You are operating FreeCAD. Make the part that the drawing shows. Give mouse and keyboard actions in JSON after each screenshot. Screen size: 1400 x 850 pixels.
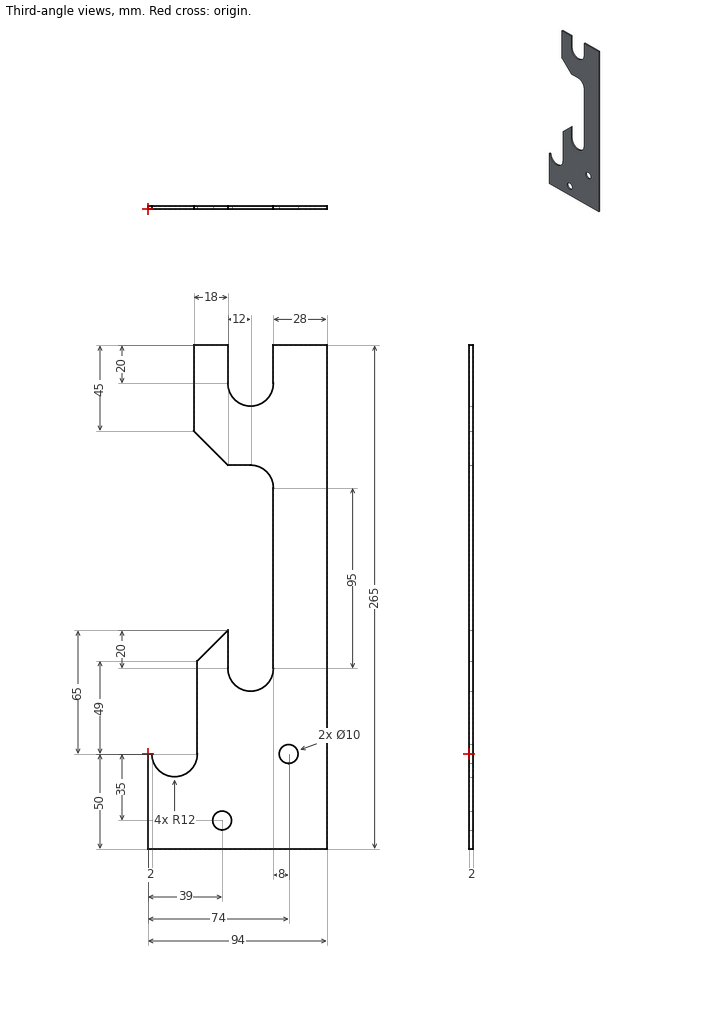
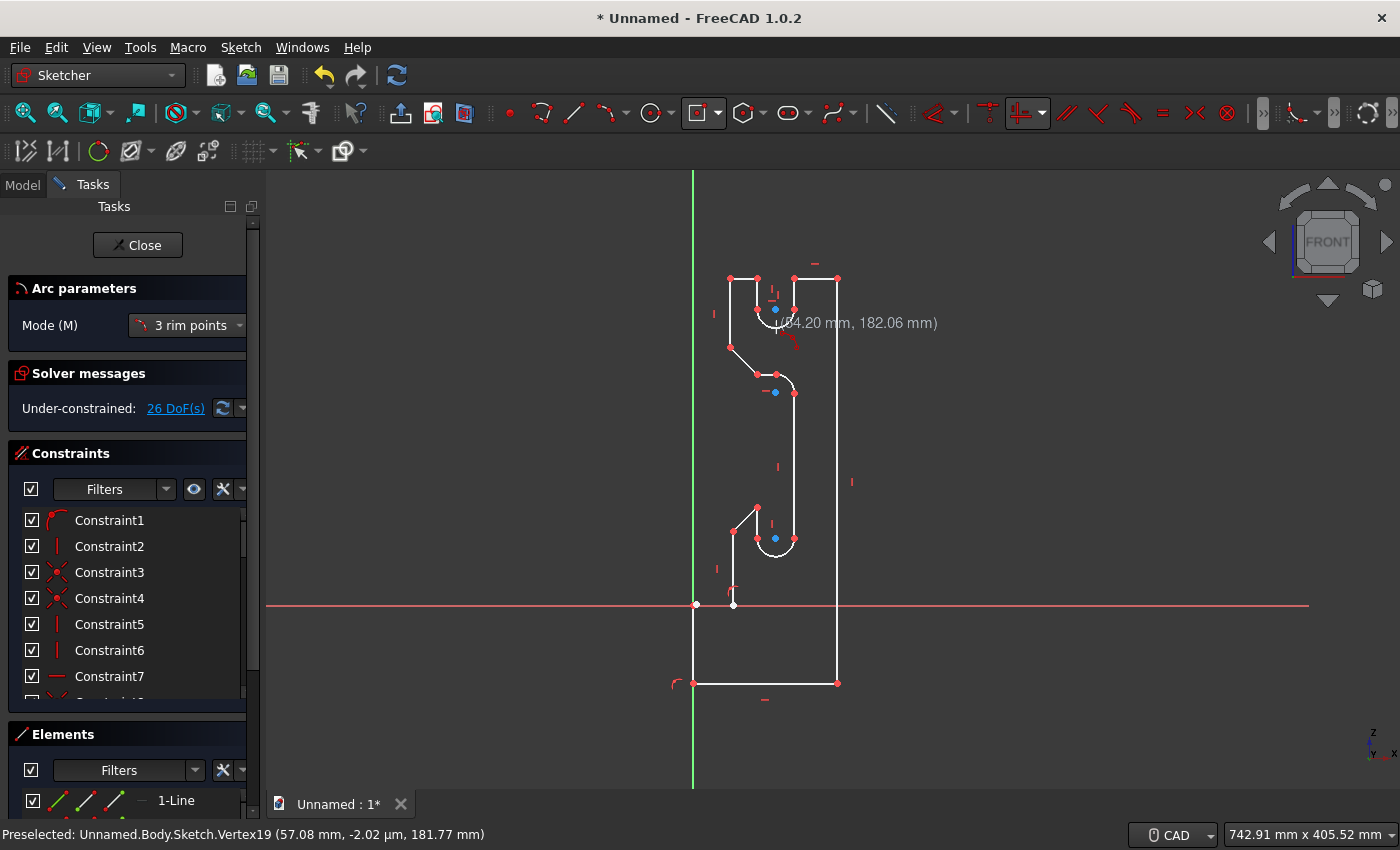
{"action": "scroll", "coordinate": [696, 606], "scroll_direction": "up", "scroll_amount": 12}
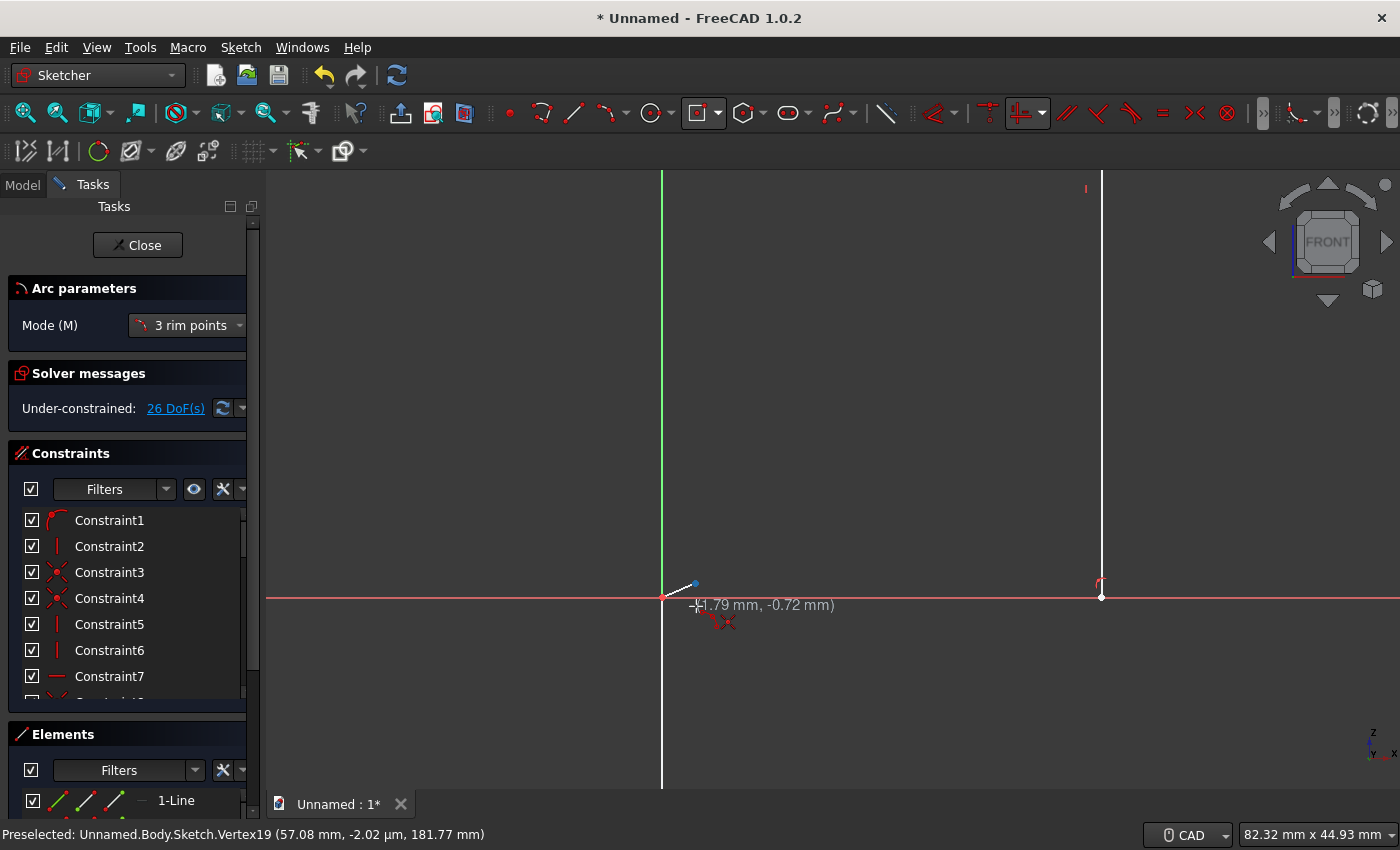
{"action": "left_click", "coordinate": [695, 583]}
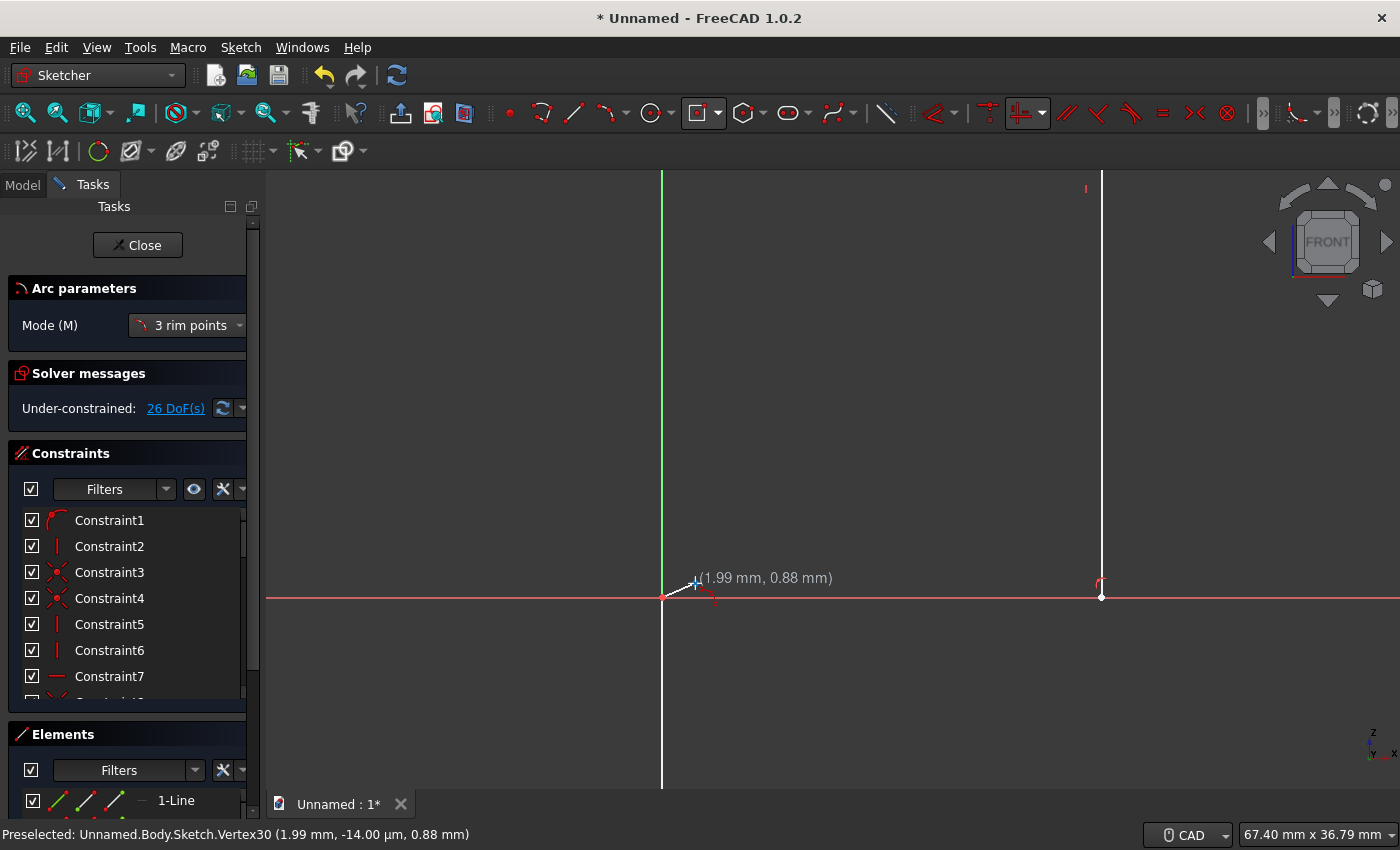
{"action": "scroll", "coordinate": [696, 606], "scroll_direction": "down", "scroll_amount": 12}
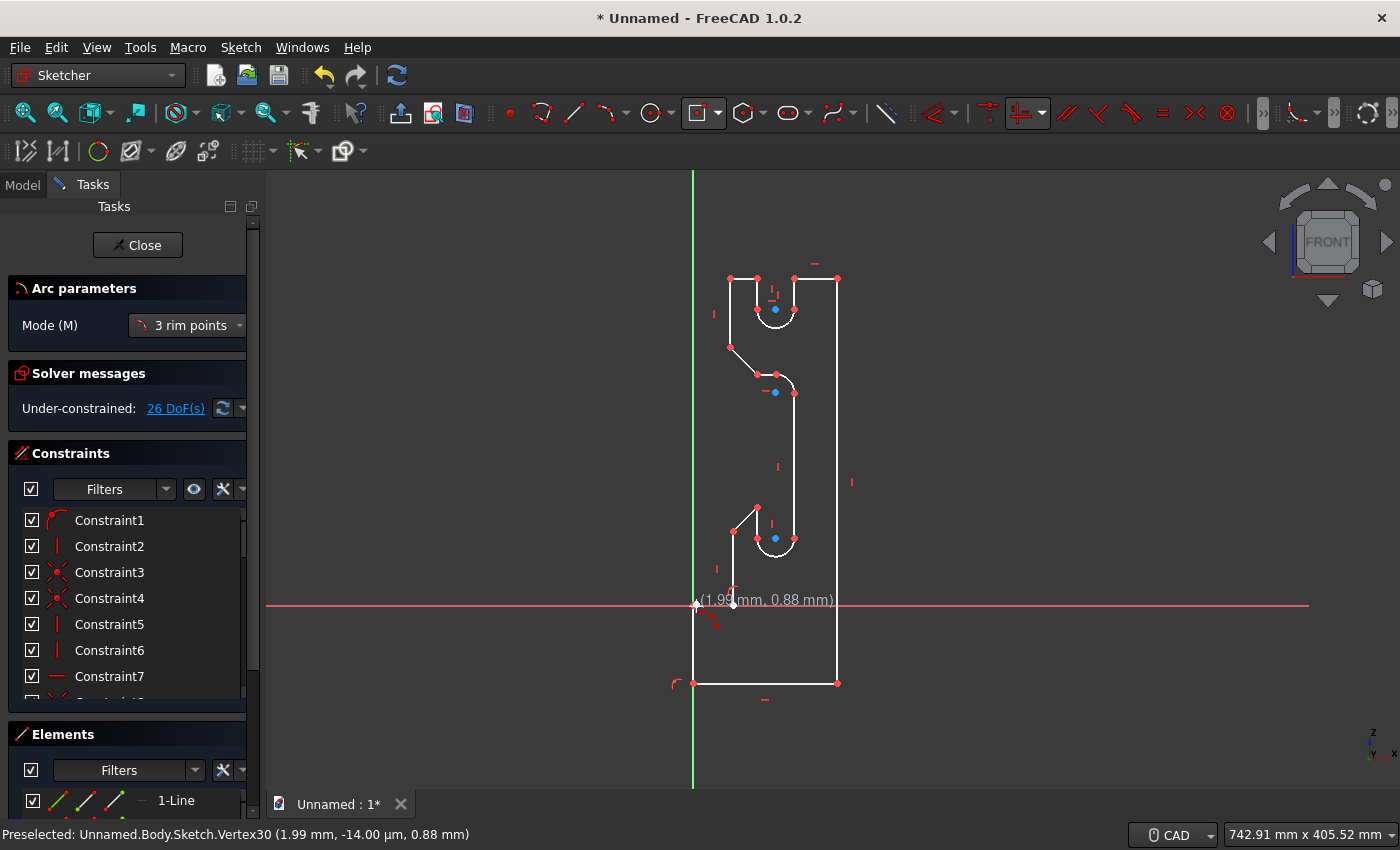
{"action": "left_click", "coordinate": [733, 606]}
{"action": "left_click", "coordinate": [715, 624]}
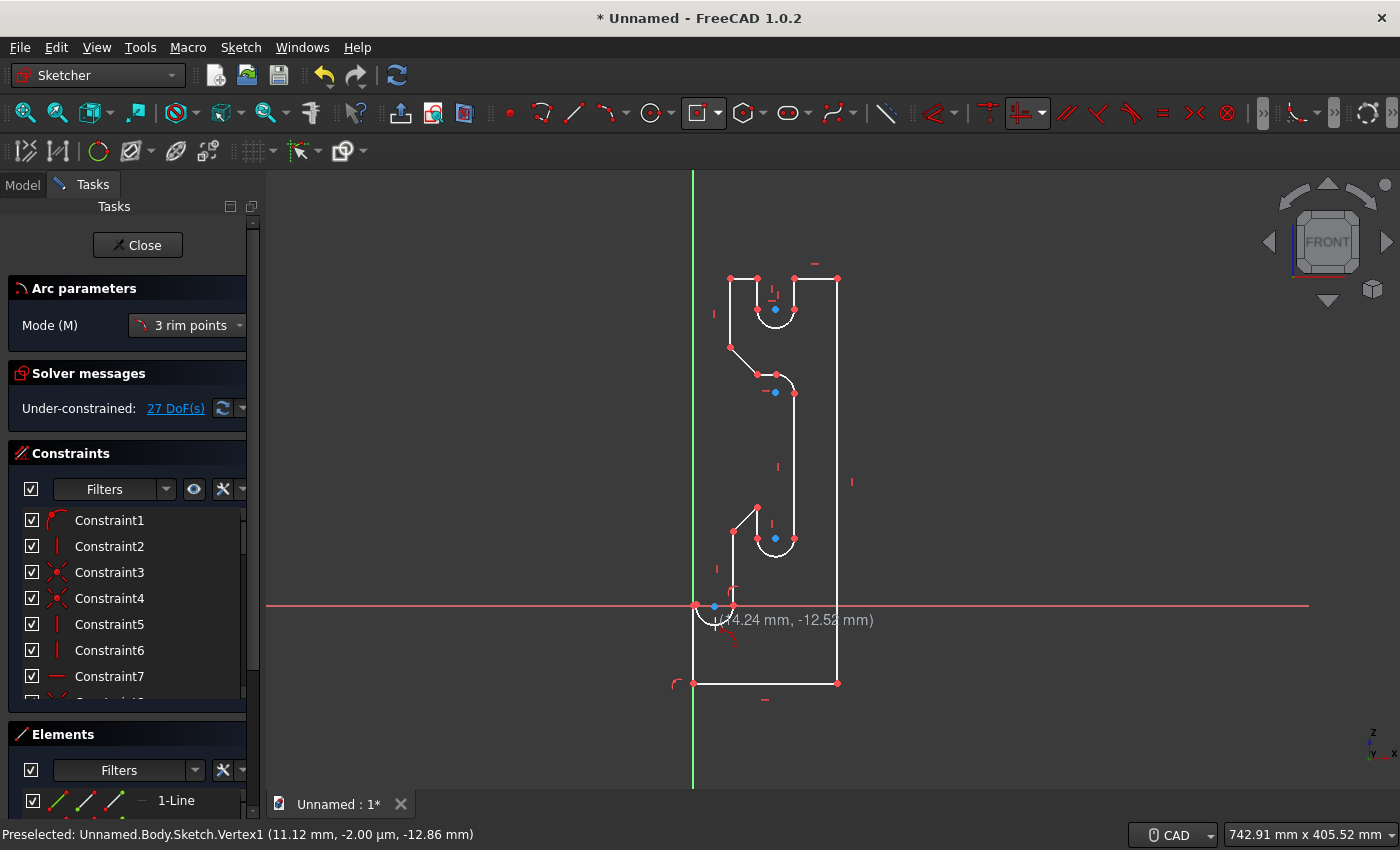
{"action": "key", "text": "g c"}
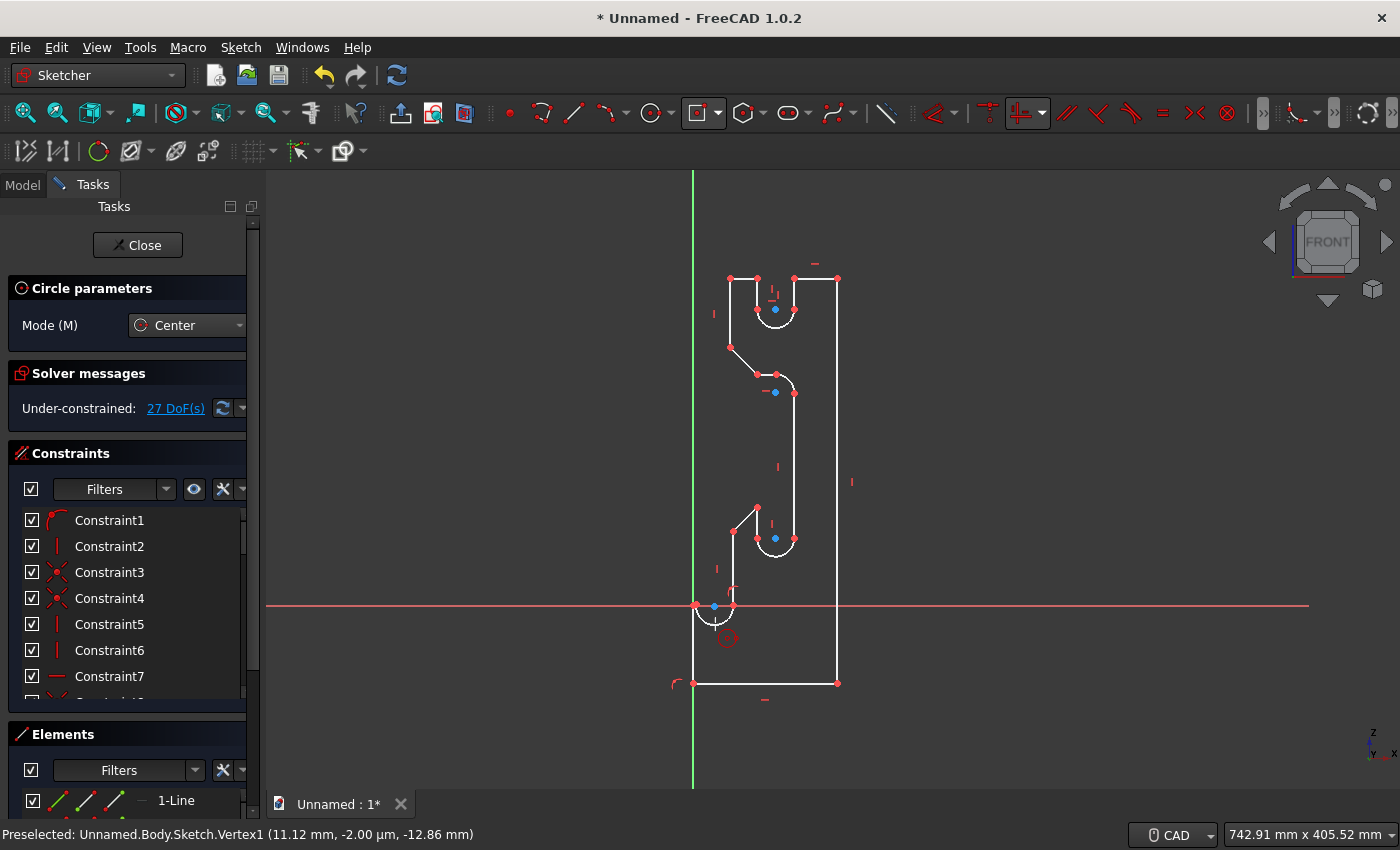
{"action": "scroll", "coordinate": [806, 606], "scroll_direction": "up", "scroll_amount": 6}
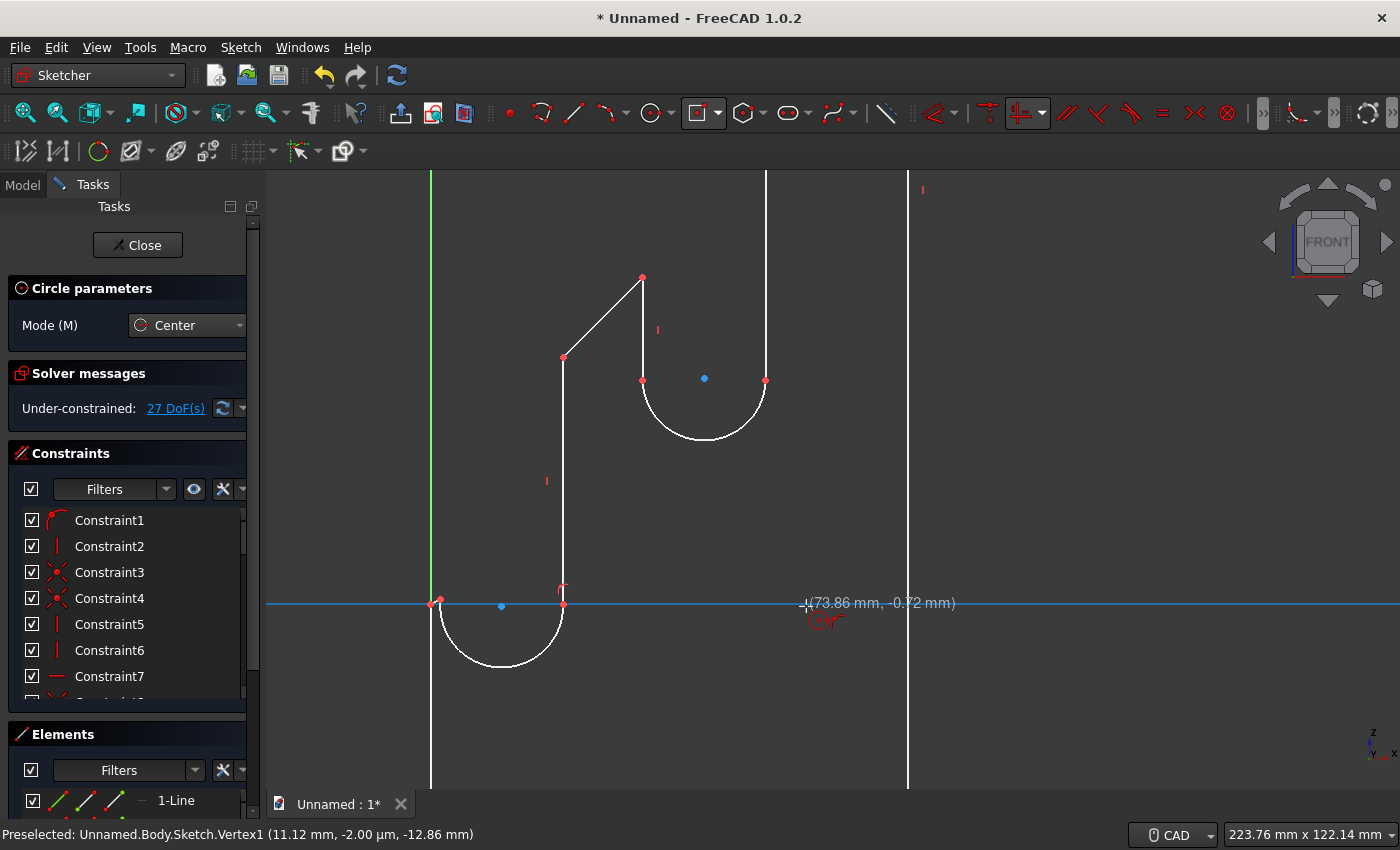
{"action": "left_click", "coordinate": [806, 604]}
{"action": "mouse_move", "coordinate": [824, 586]}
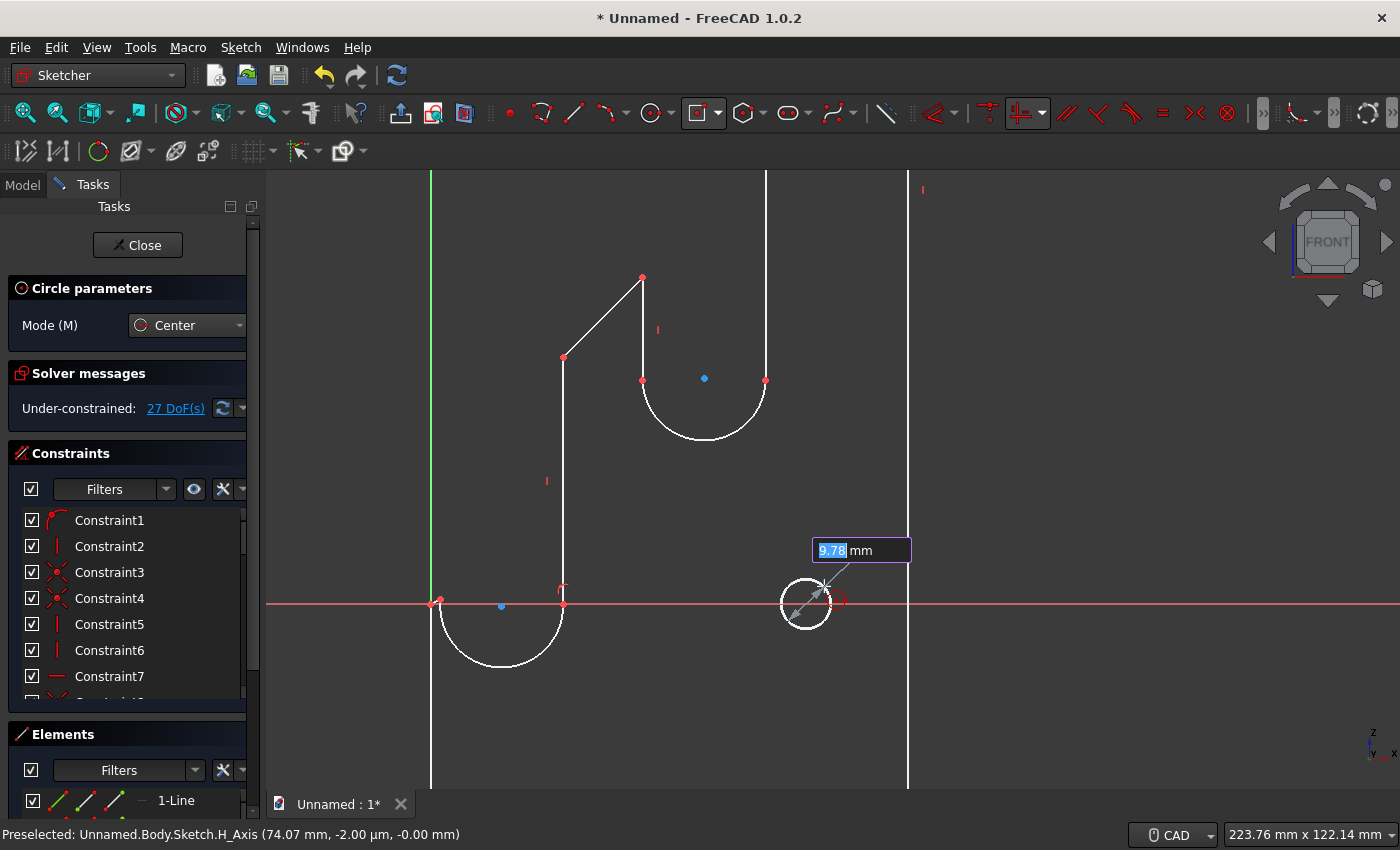
{"action": "type", "text": "10"}
{"action": "key", "text": "Return"}